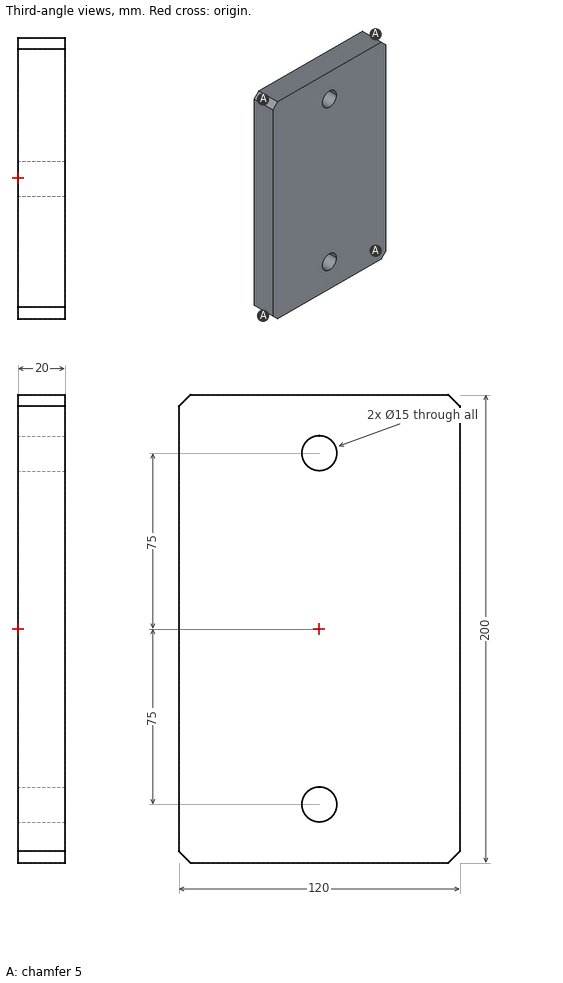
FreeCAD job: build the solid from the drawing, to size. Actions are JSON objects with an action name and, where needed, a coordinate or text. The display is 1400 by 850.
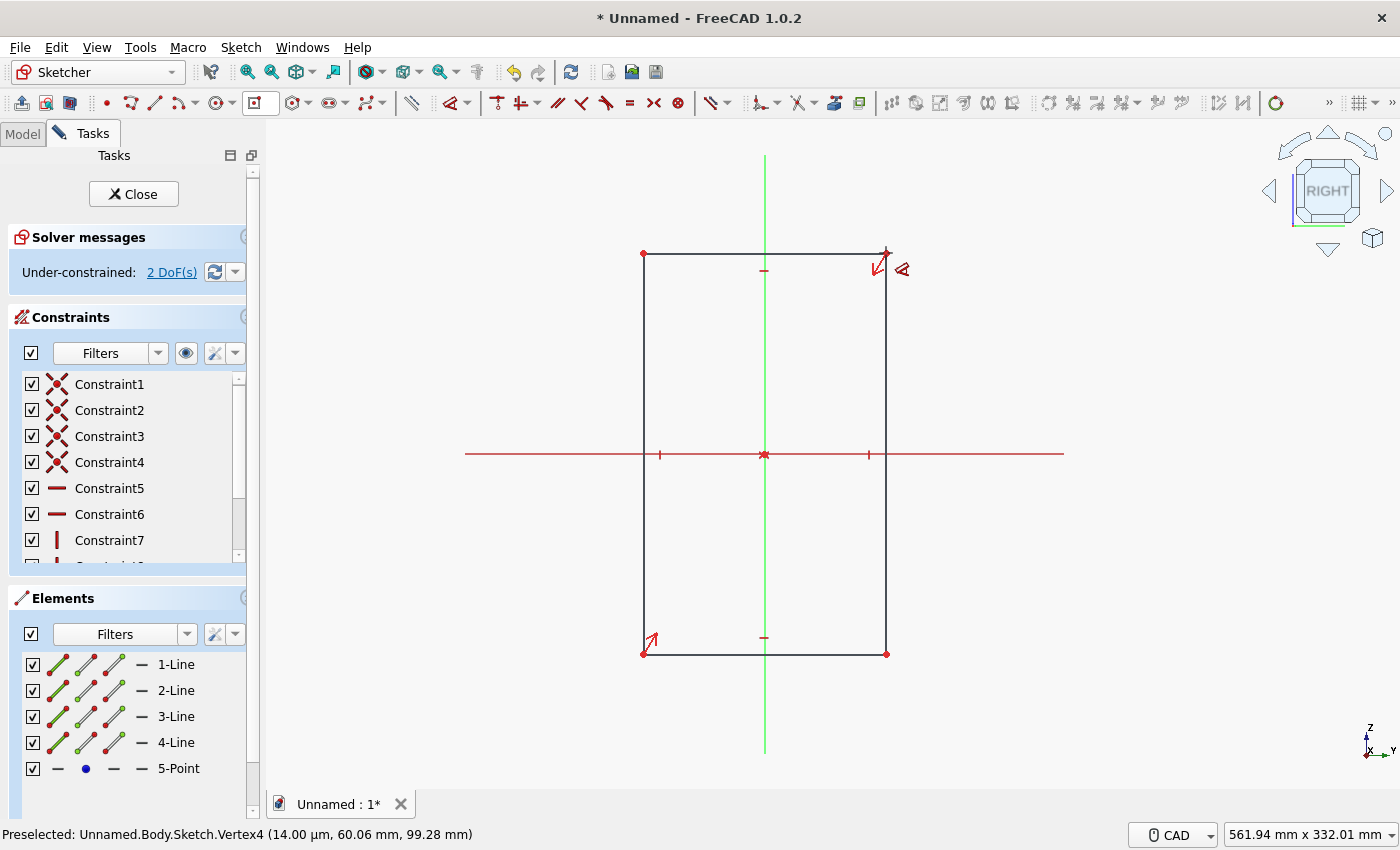
{"action": "left_click", "coordinate": [716, 655]}
{"action": "left_click", "coordinate": [709, 689]}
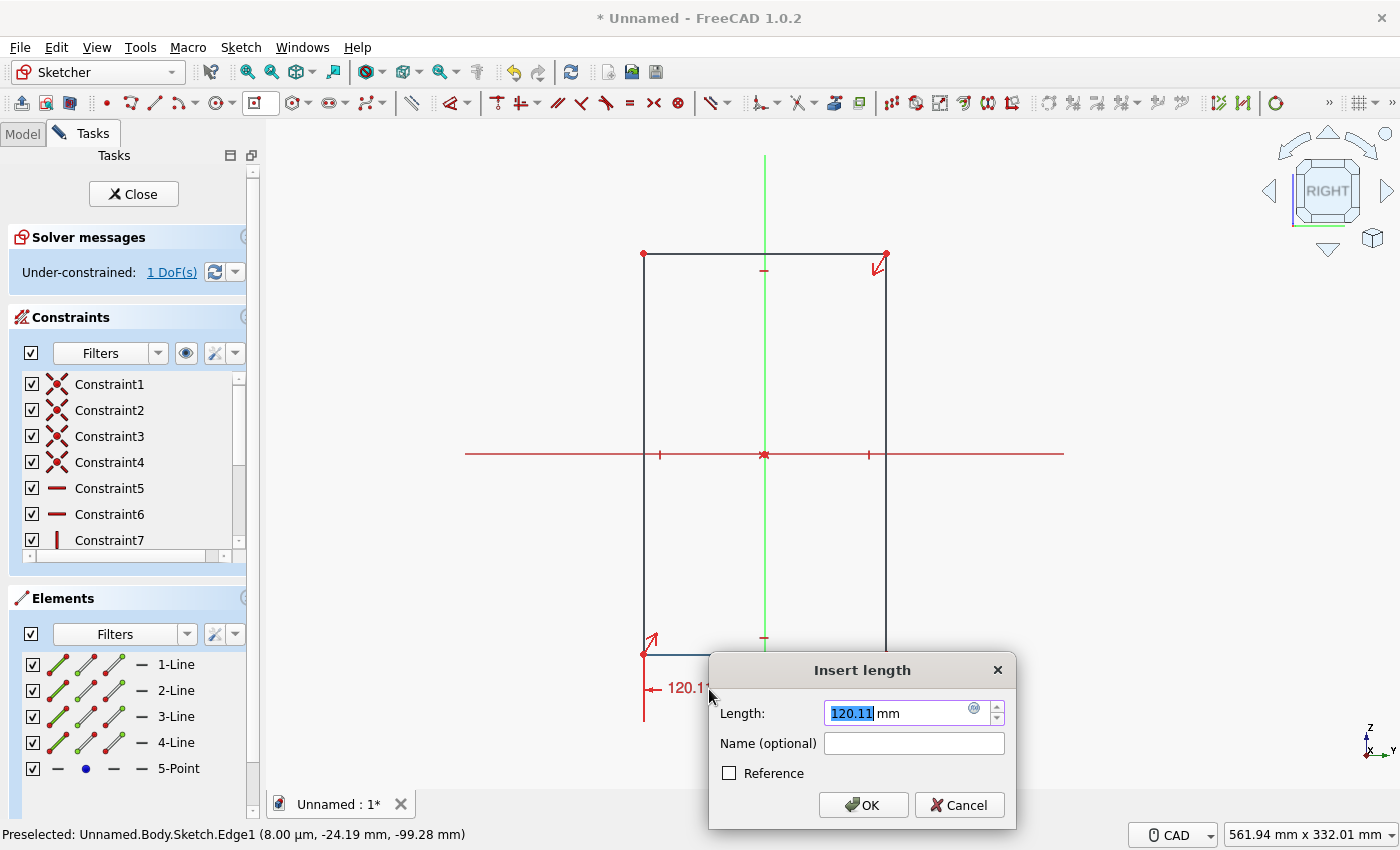
{"action": "type", "text": "120"}
{"action": "key", "text": "Return"}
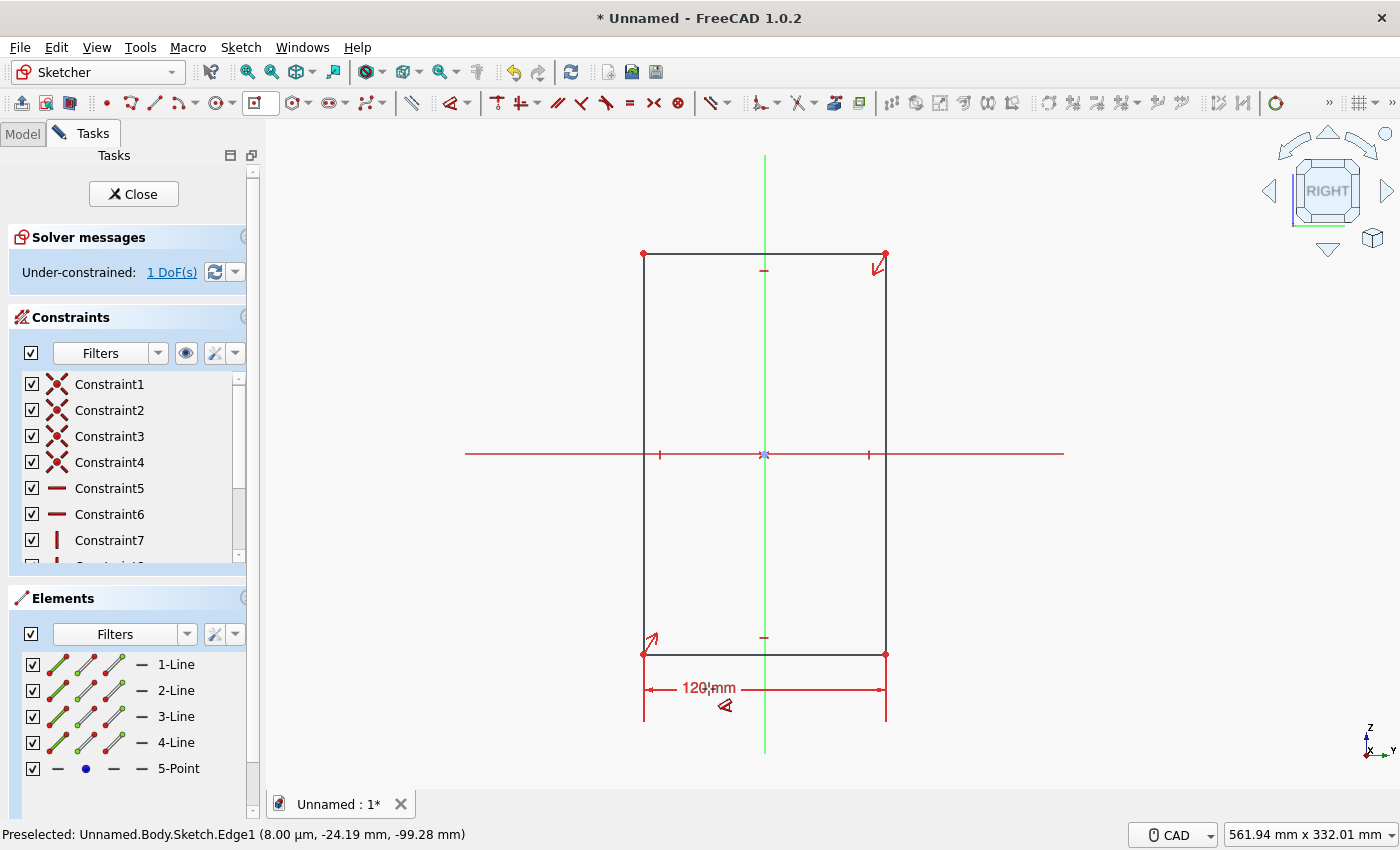
{"action": "left_click", "coordinate": [886, 534]}
{"action": "left_click", "coordinate": [920, 362]}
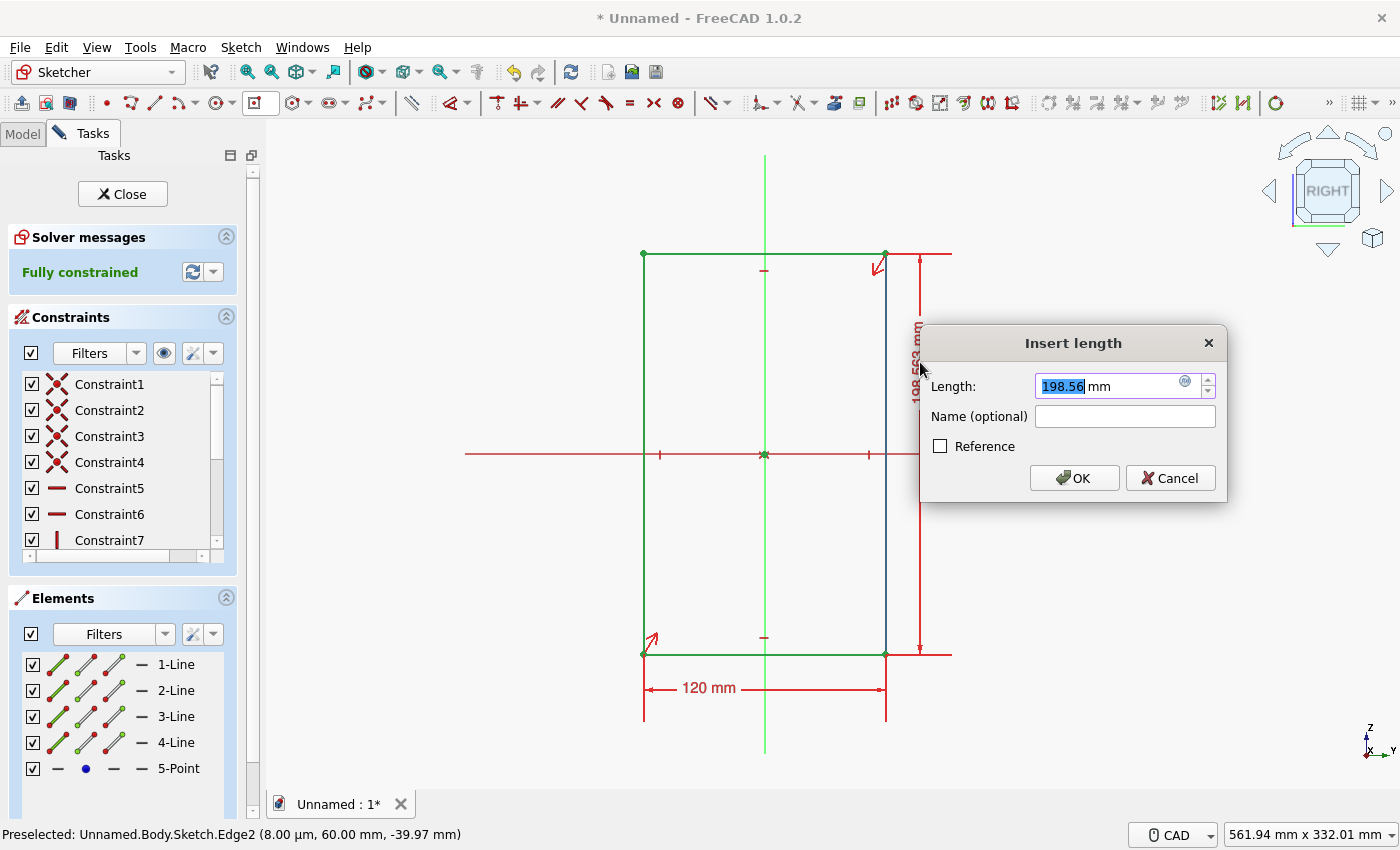
{"action": "type", "text": "200"}
{"action": "key", "text": "Return"}
{"action": "key", "text": "Escape"}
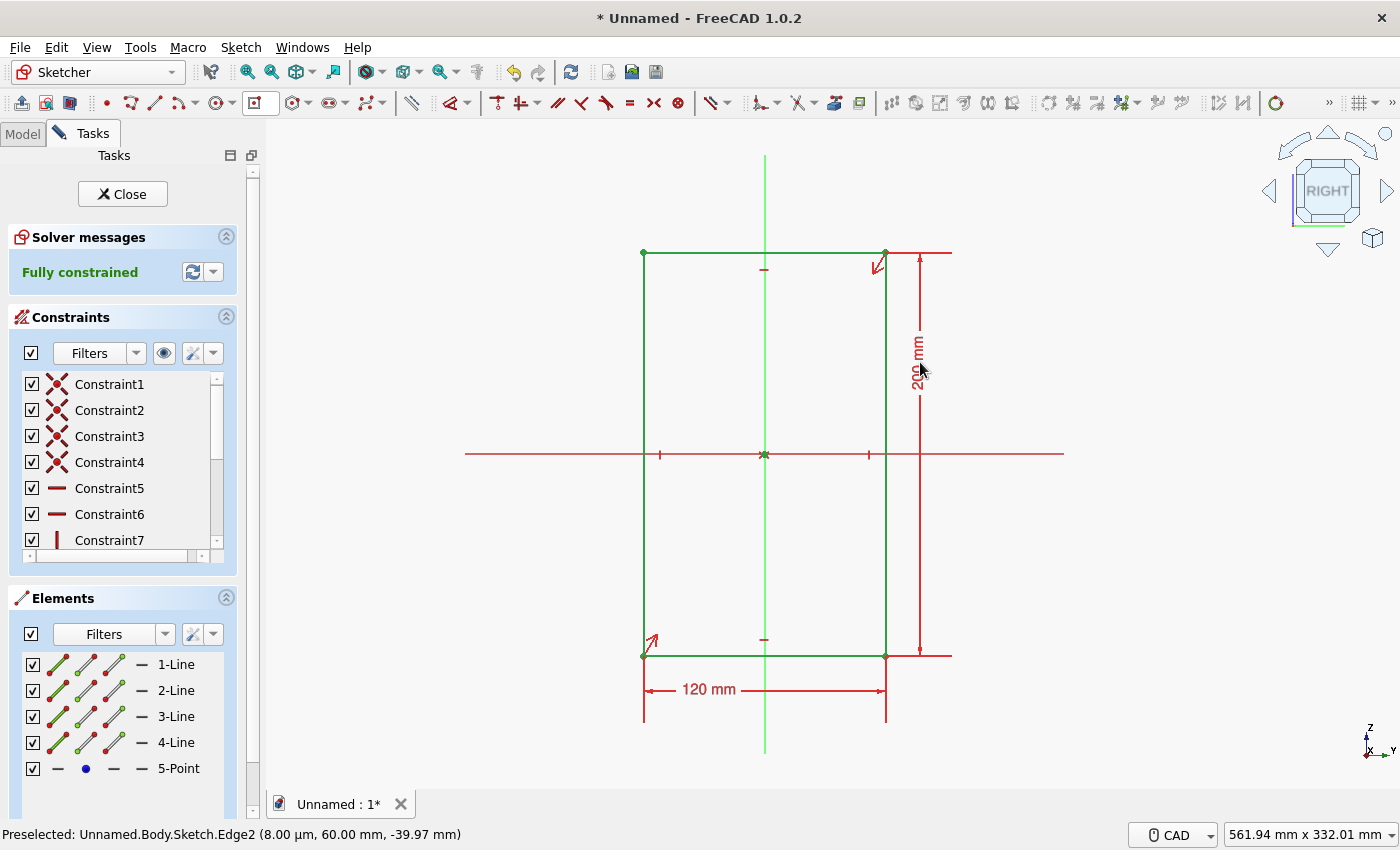
{"action": "left_click", "coordinate": [123, 194]}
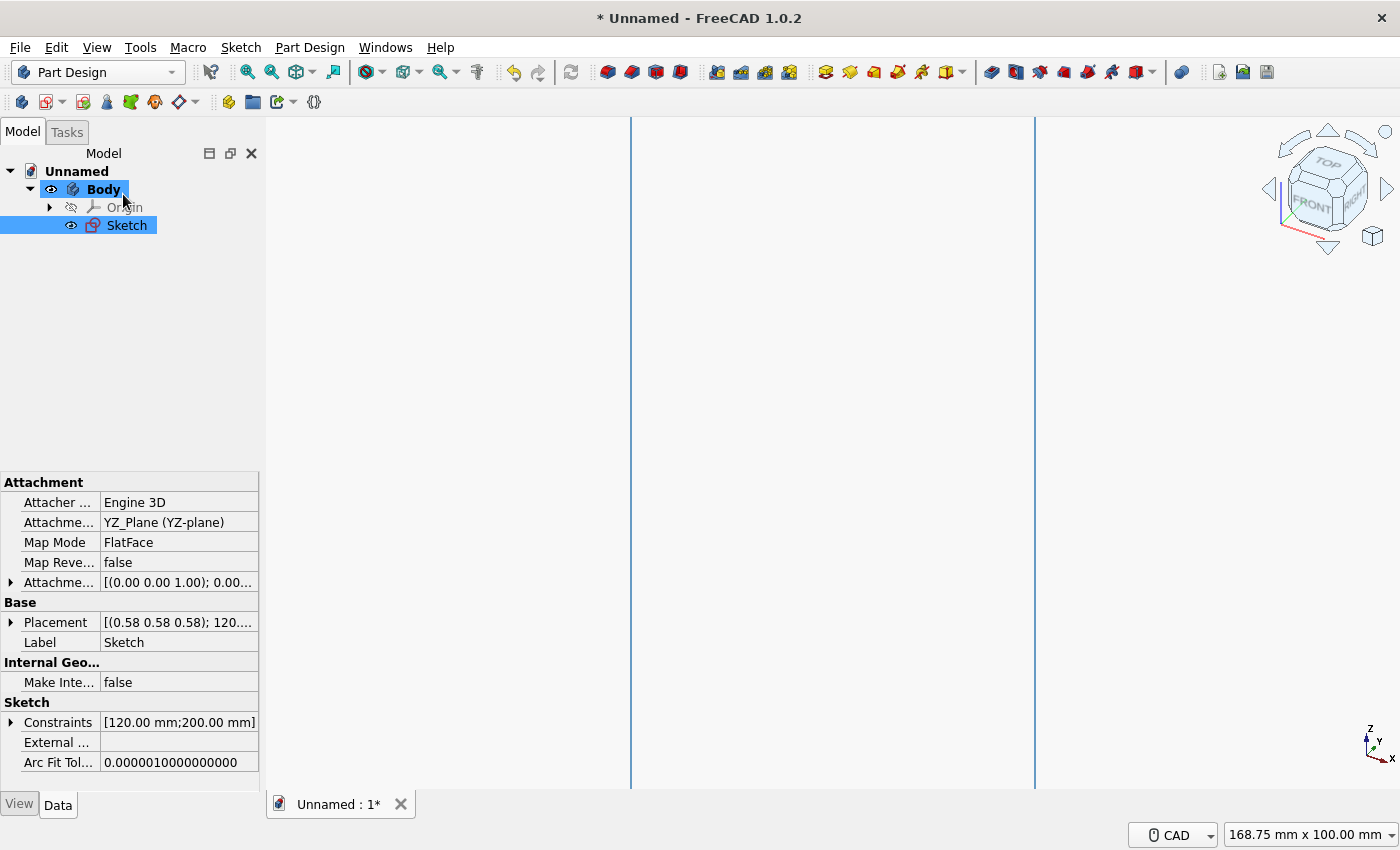
{"action": "left_click", "coordinate": [826, 72]}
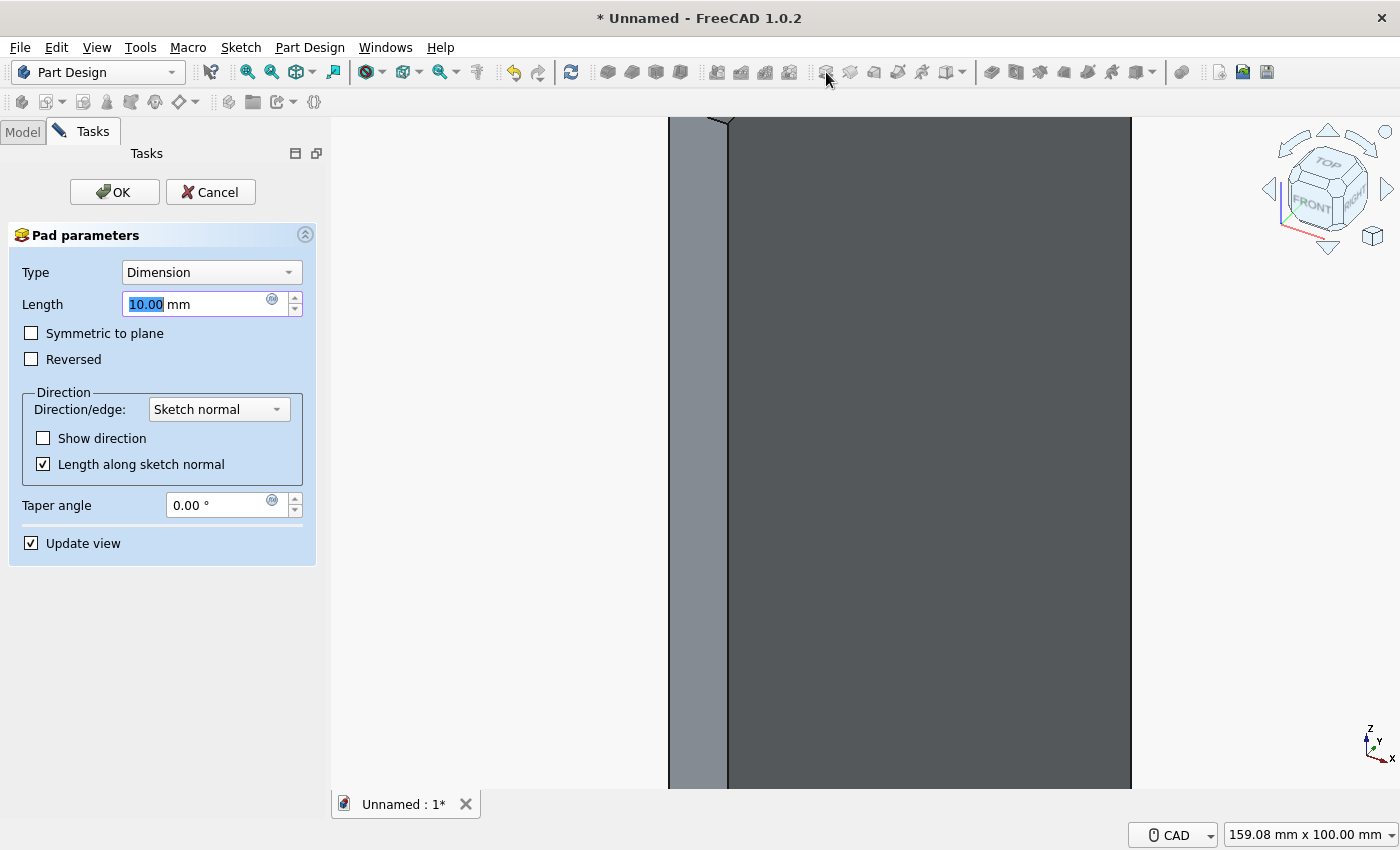
{"action": "type", "text": "20"}
{"action": "key", "text": "Tab"}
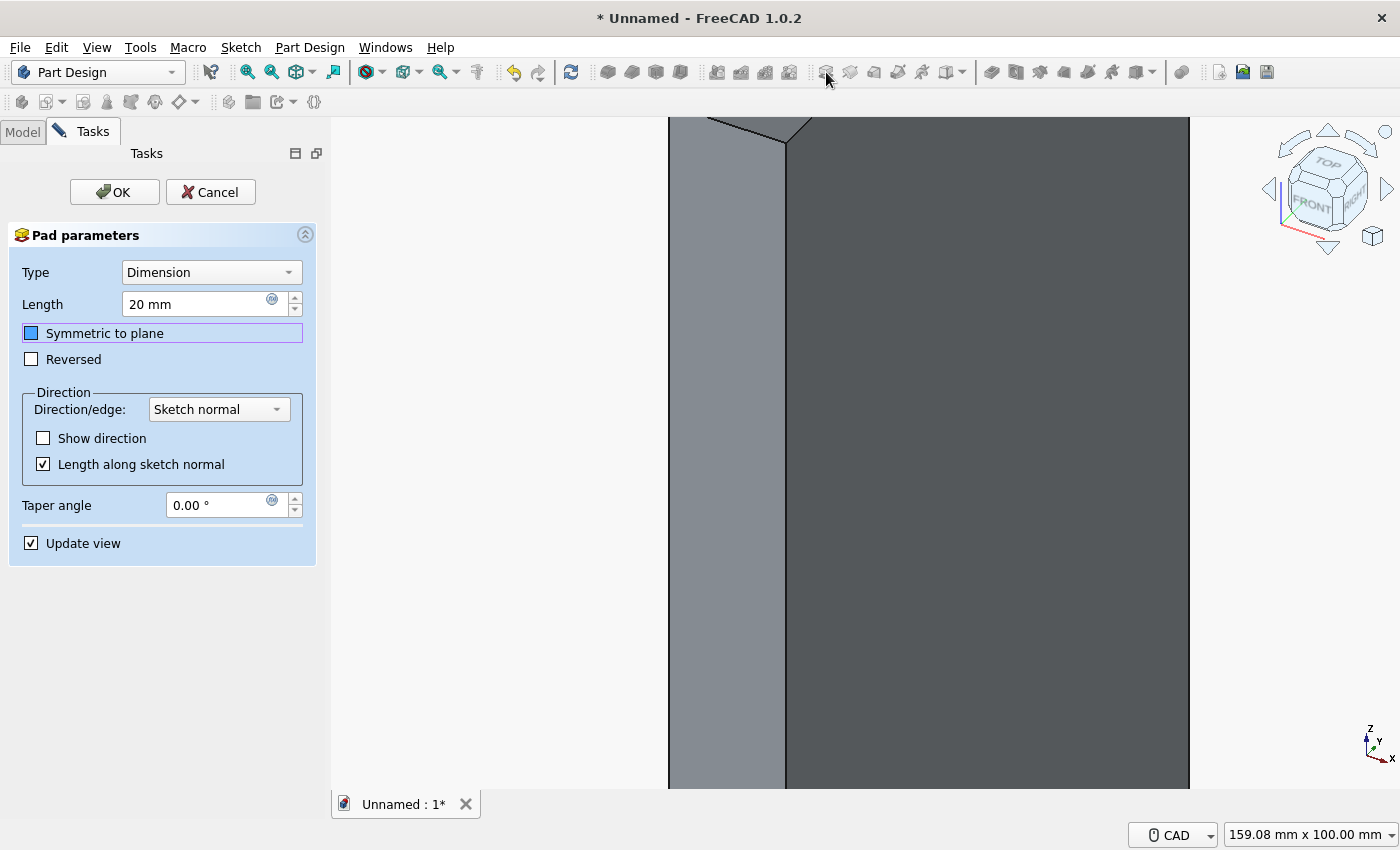
{"action": "left_click", "coordinate": [115, 192]}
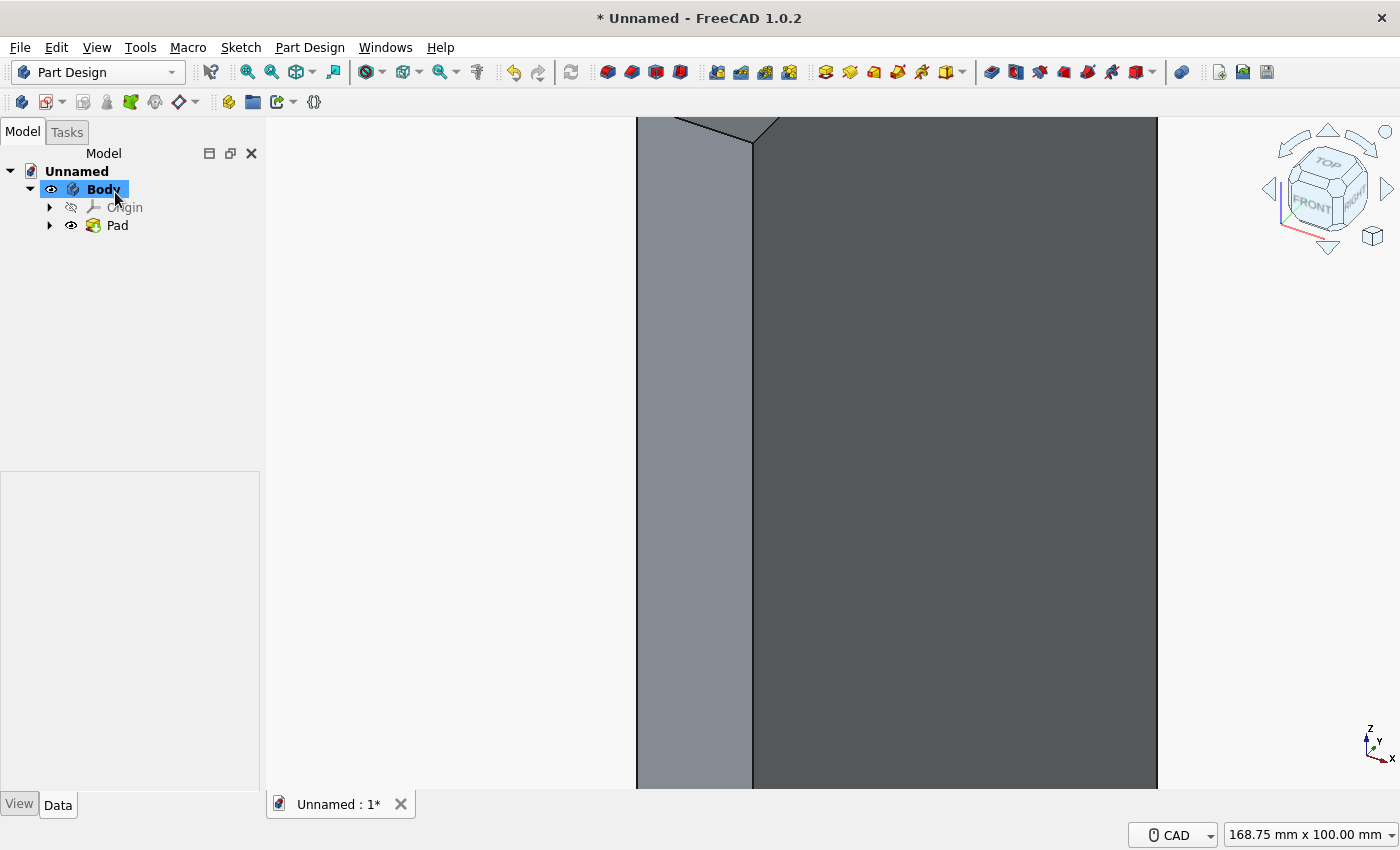
{"action": "key", "text": "v f"}